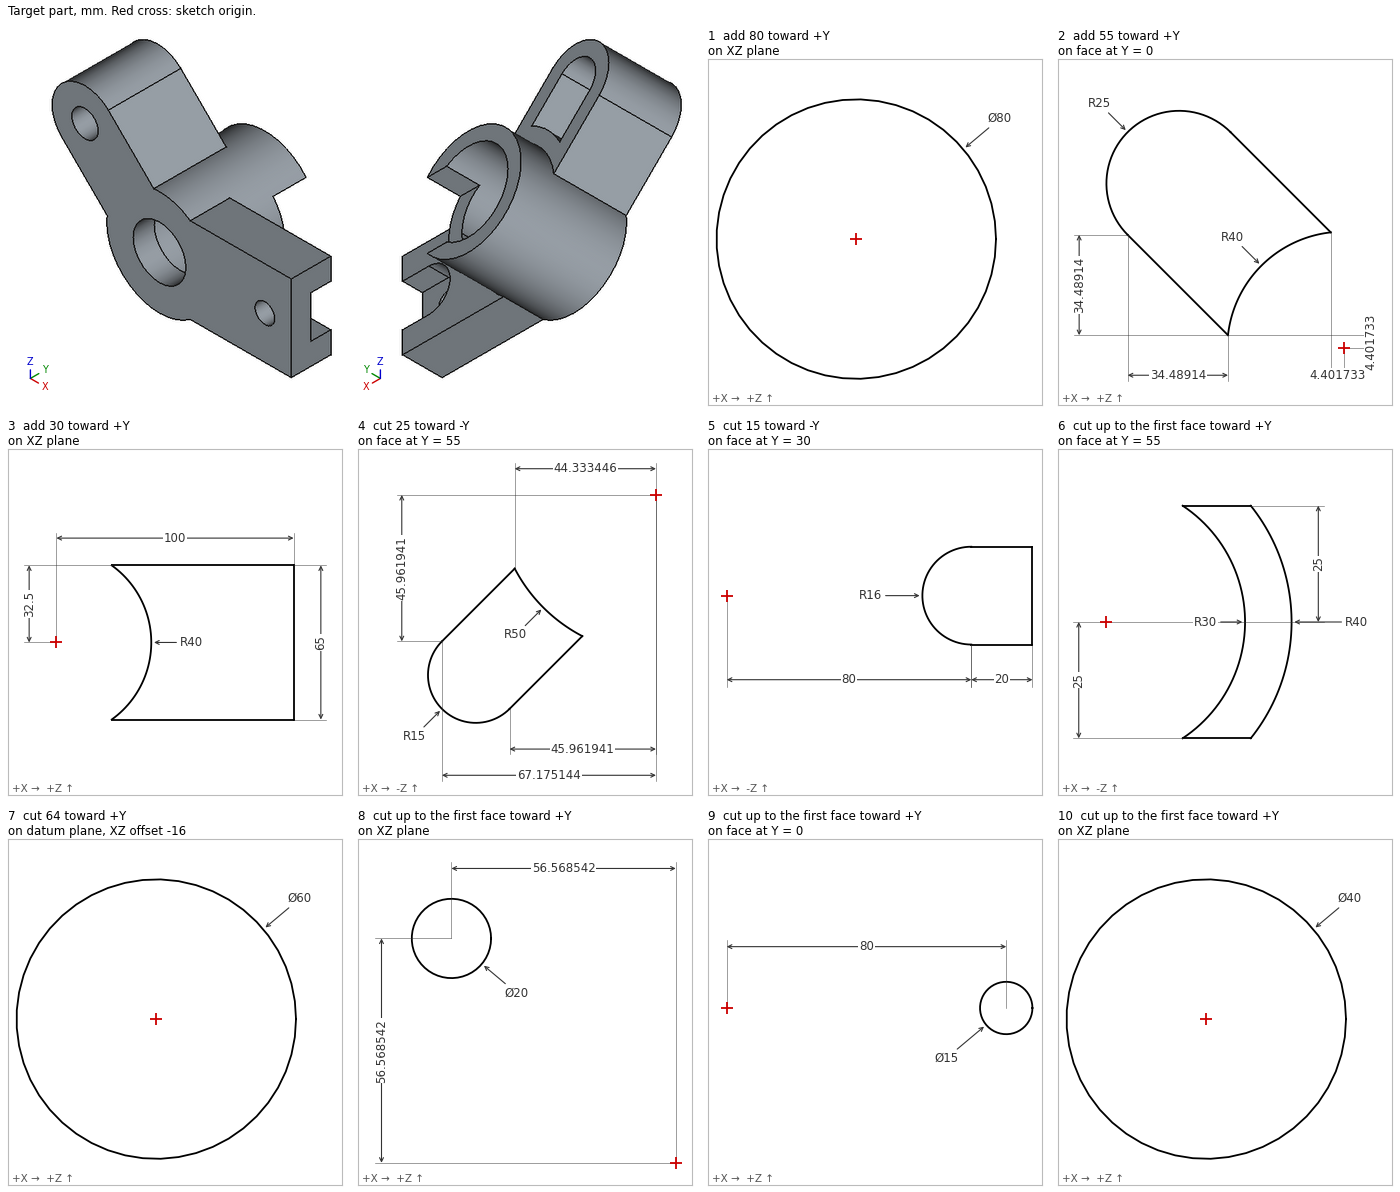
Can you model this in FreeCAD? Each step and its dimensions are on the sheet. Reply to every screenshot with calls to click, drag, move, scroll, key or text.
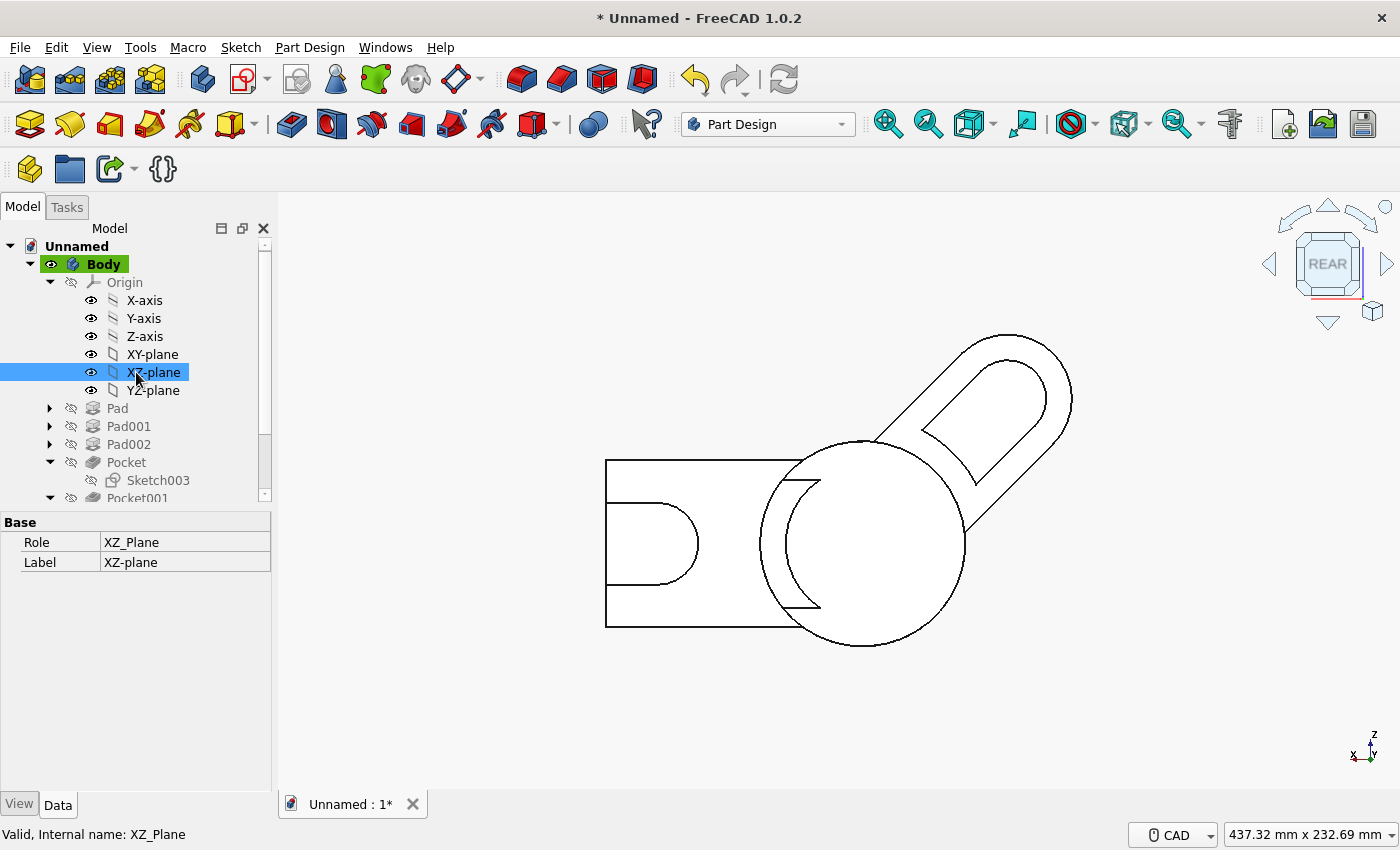
click(456, 80)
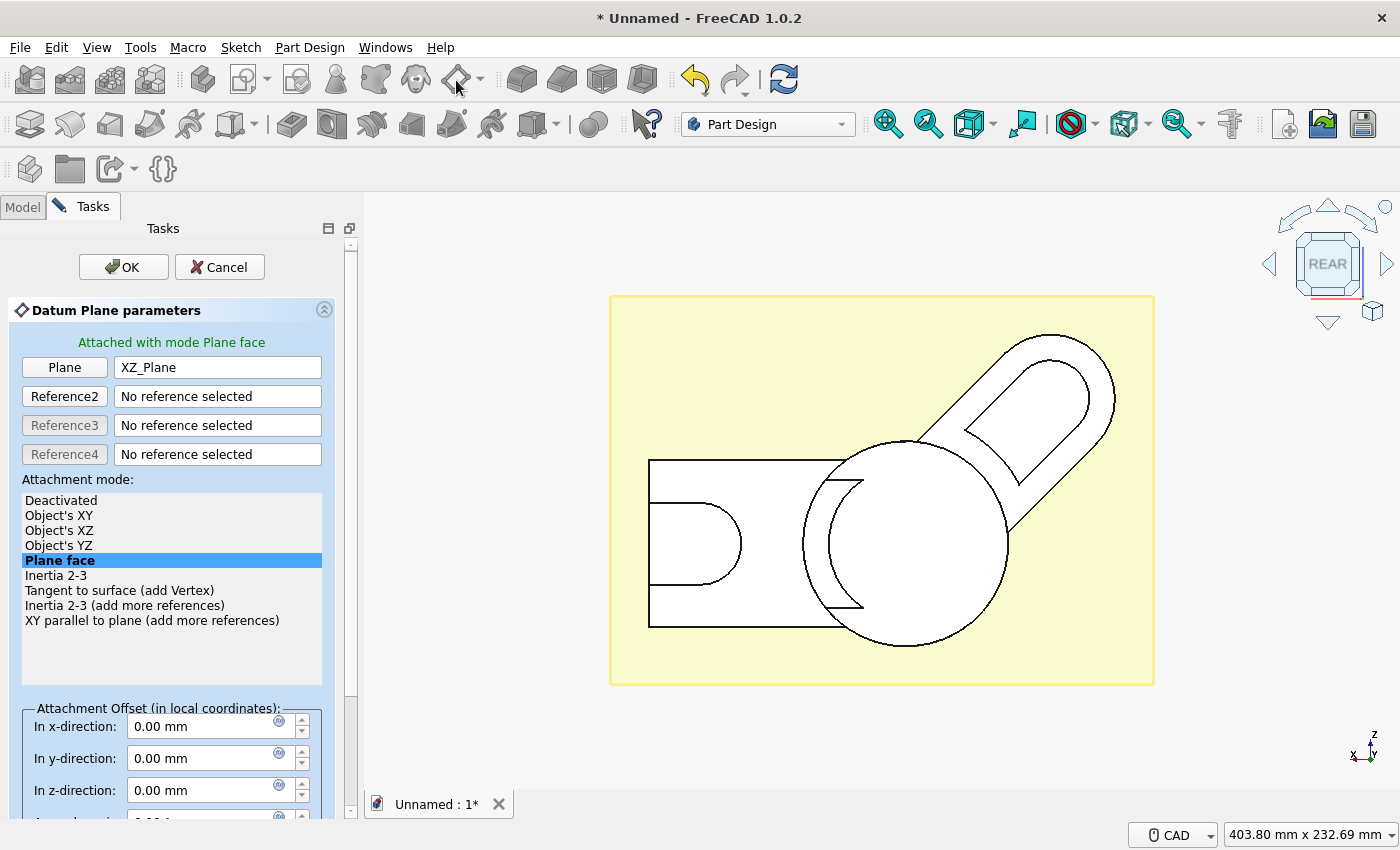
triple_click(210, 790)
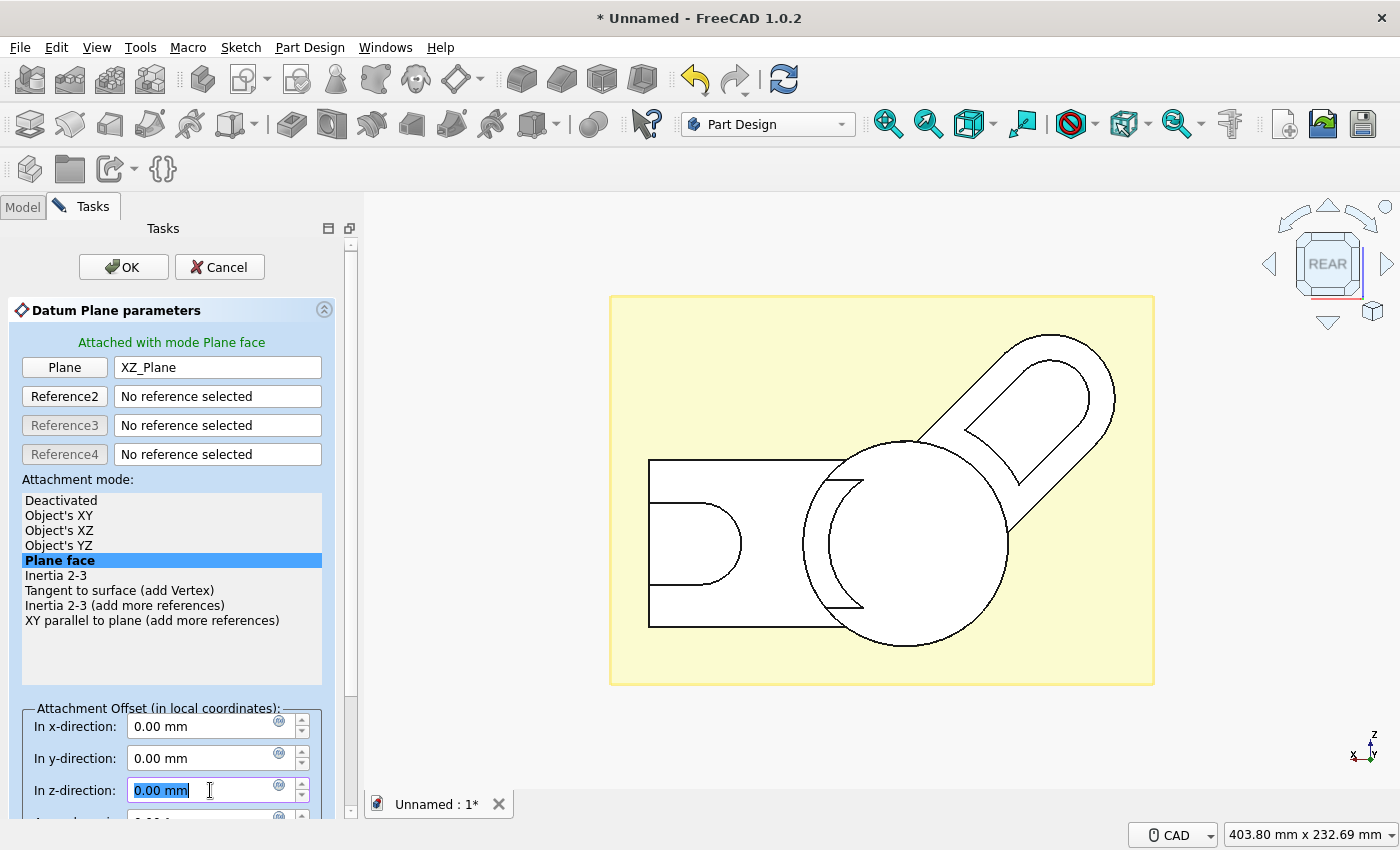
text(-16)
key(Tab)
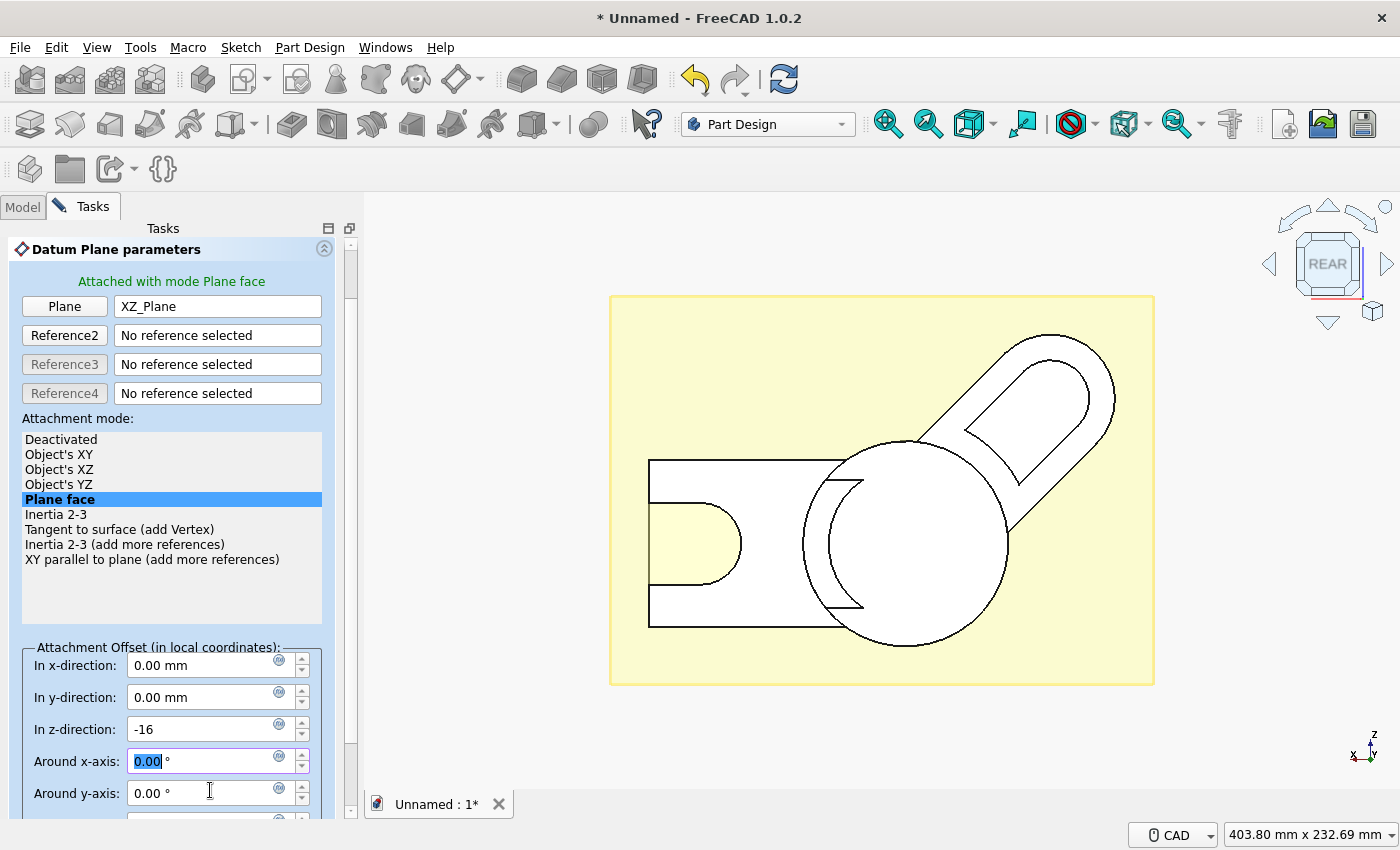
scroll(351, 528, up, 2)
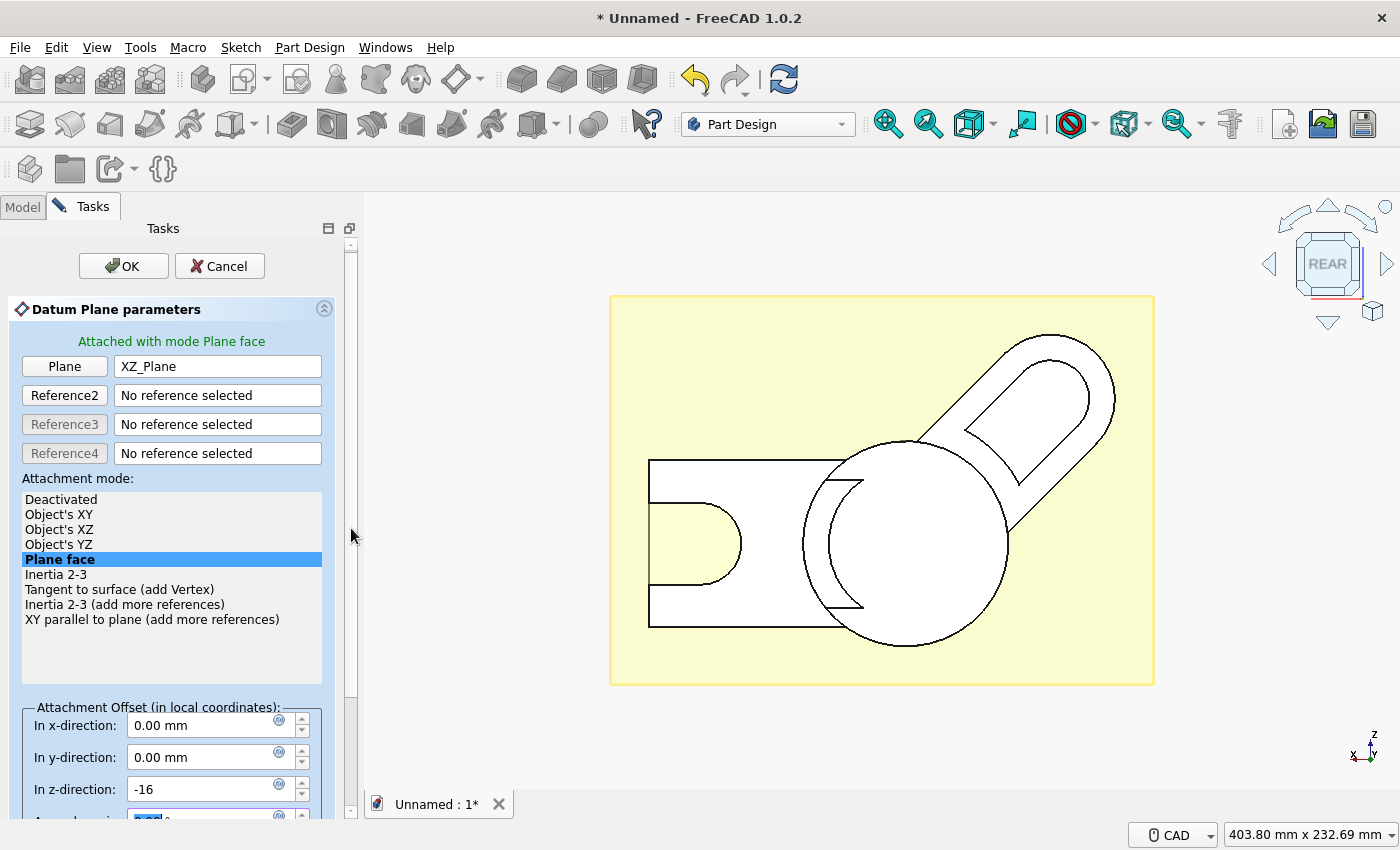
click(124, 267)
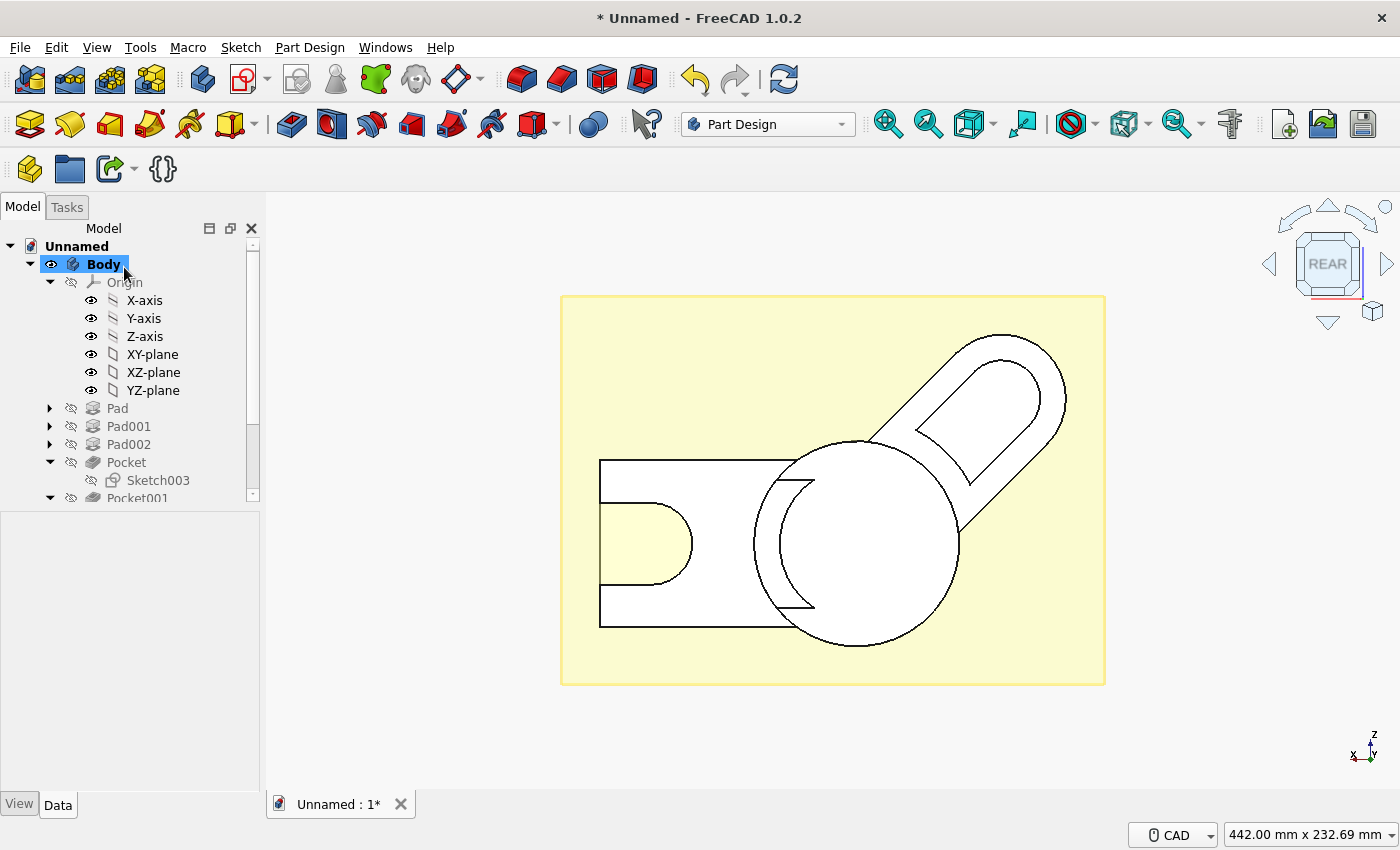
scroll(100, 368, down, 3)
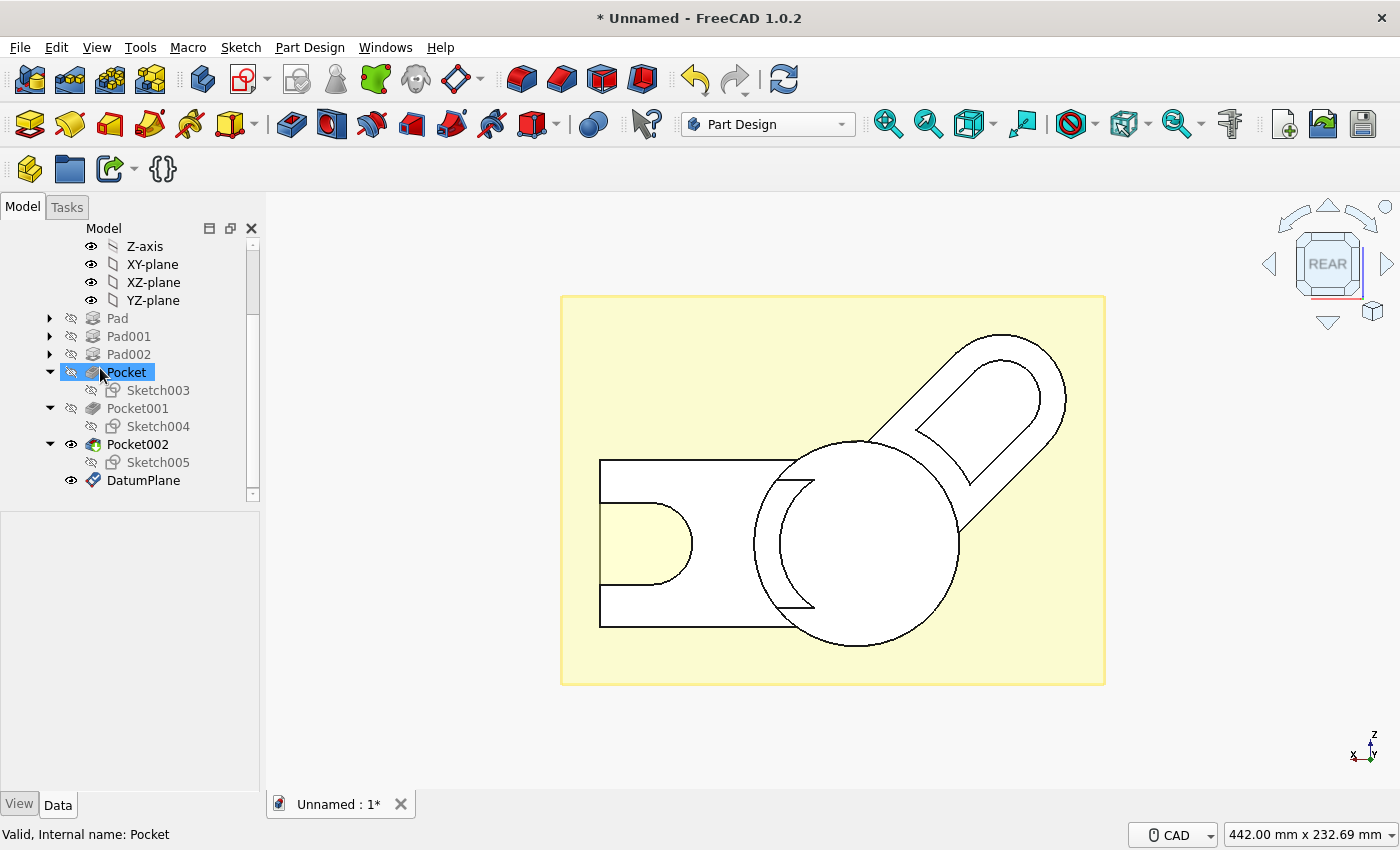
click(116, 480)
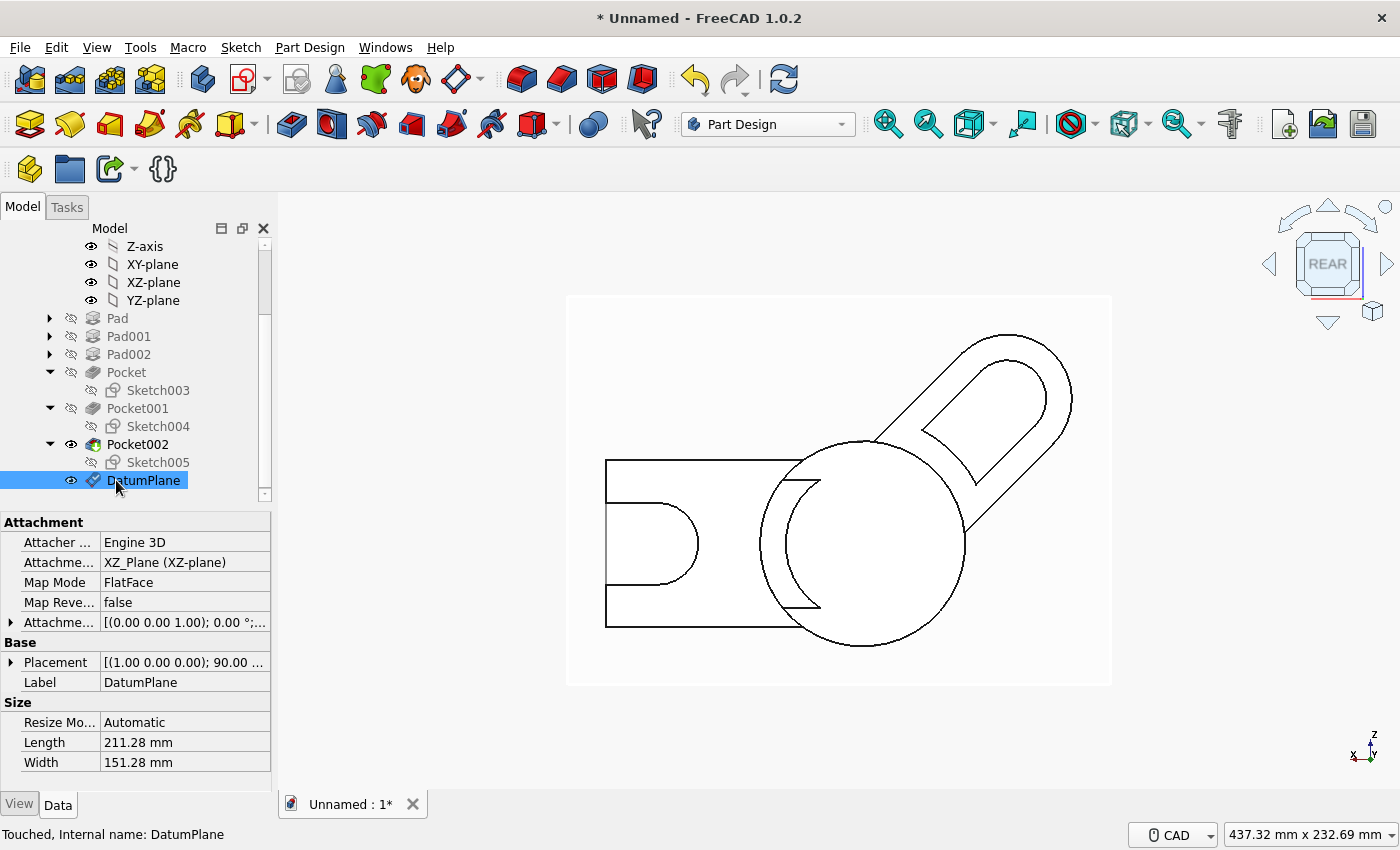
click(244, 80)